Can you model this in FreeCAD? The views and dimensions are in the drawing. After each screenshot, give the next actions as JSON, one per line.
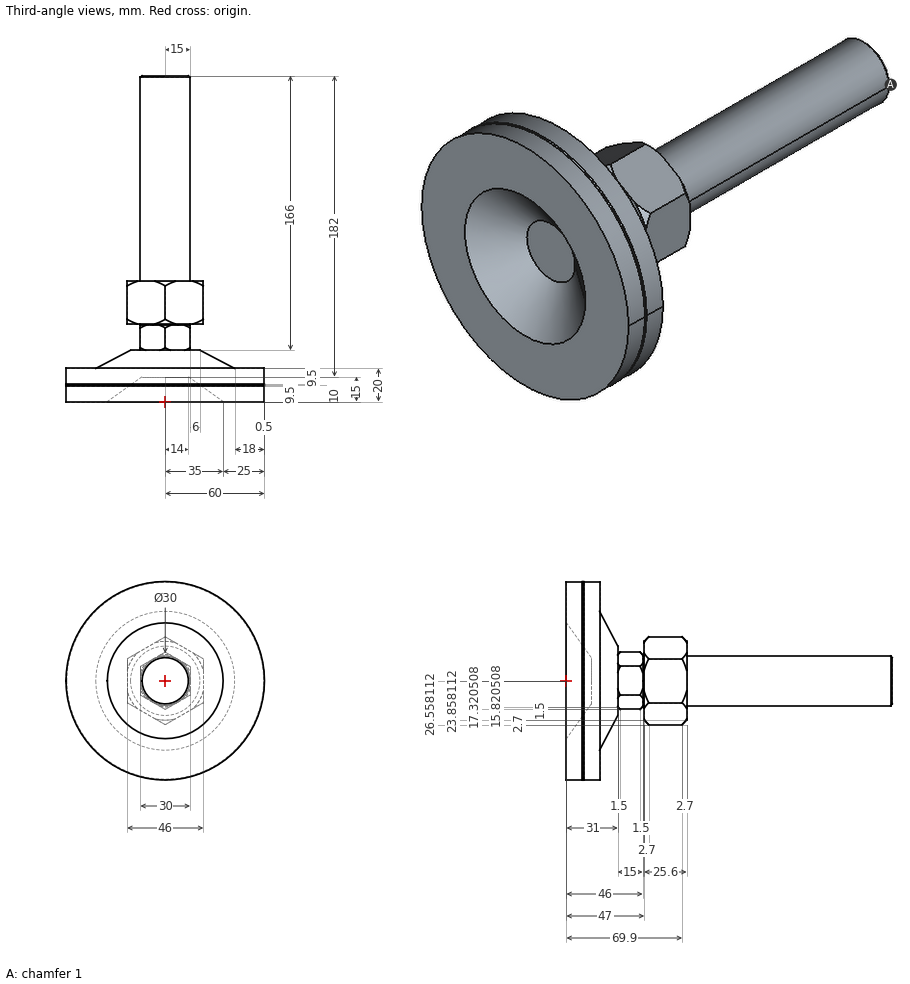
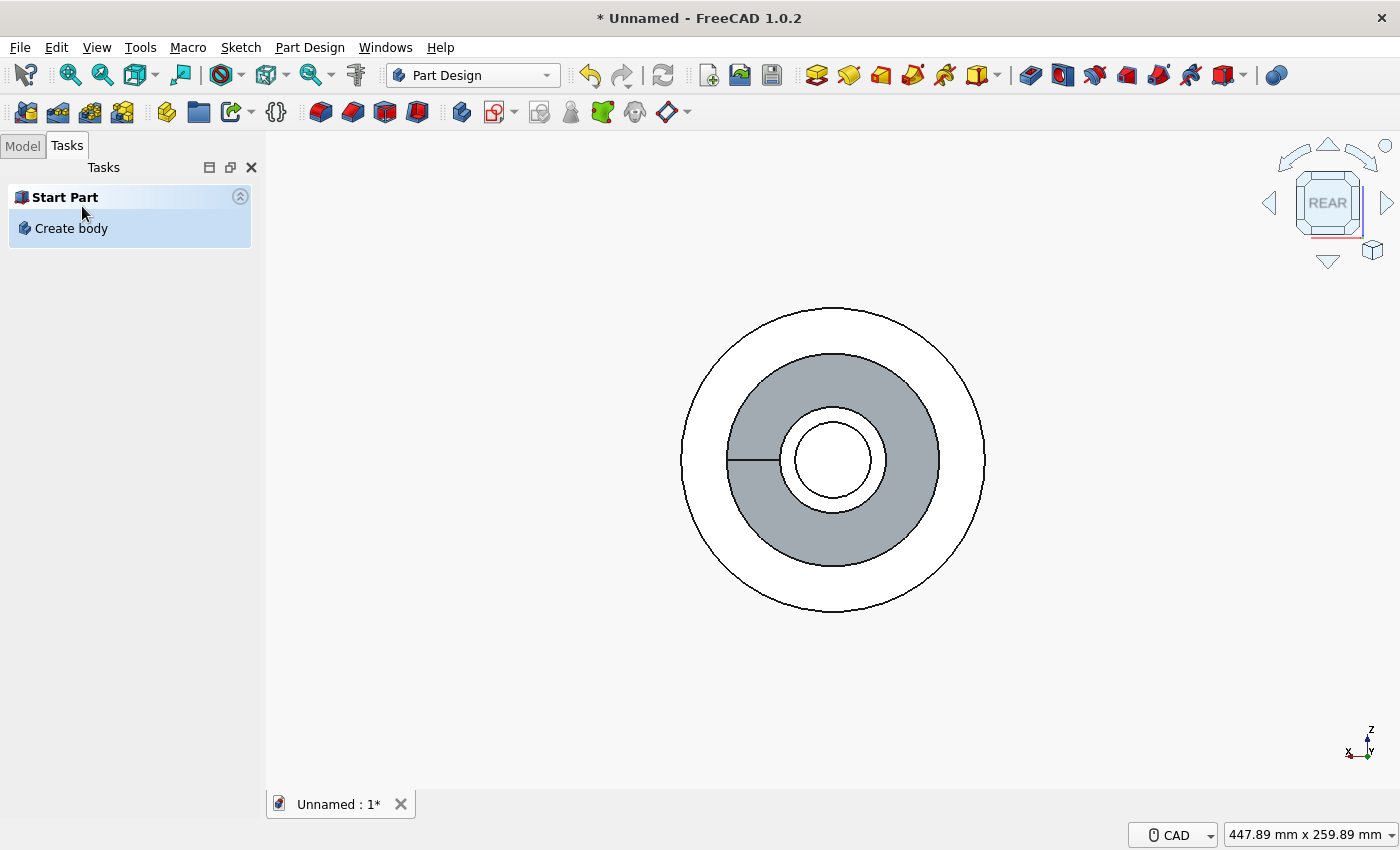
{"action": "key", "text": "2"}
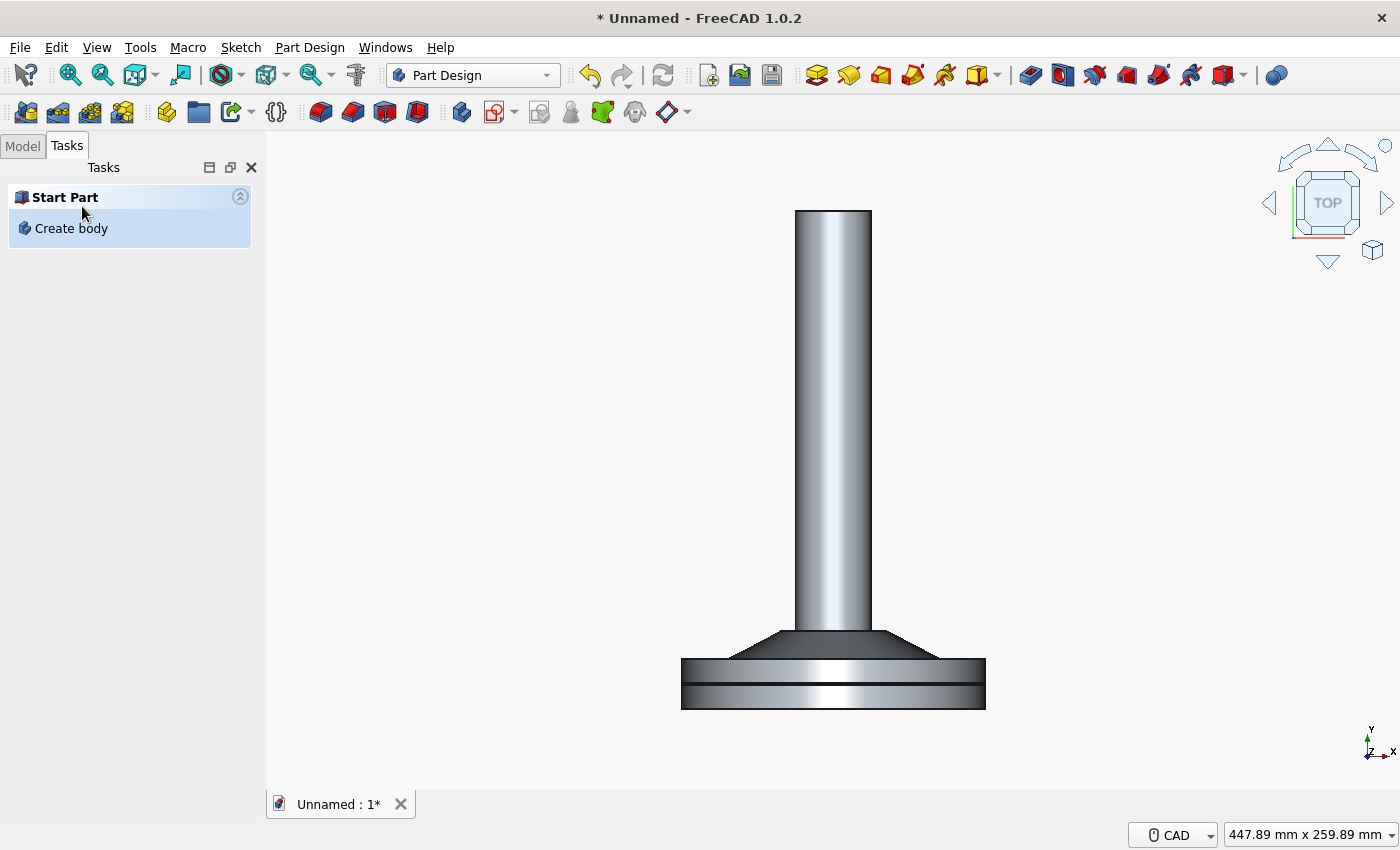
{"action": "key", "text": "3"}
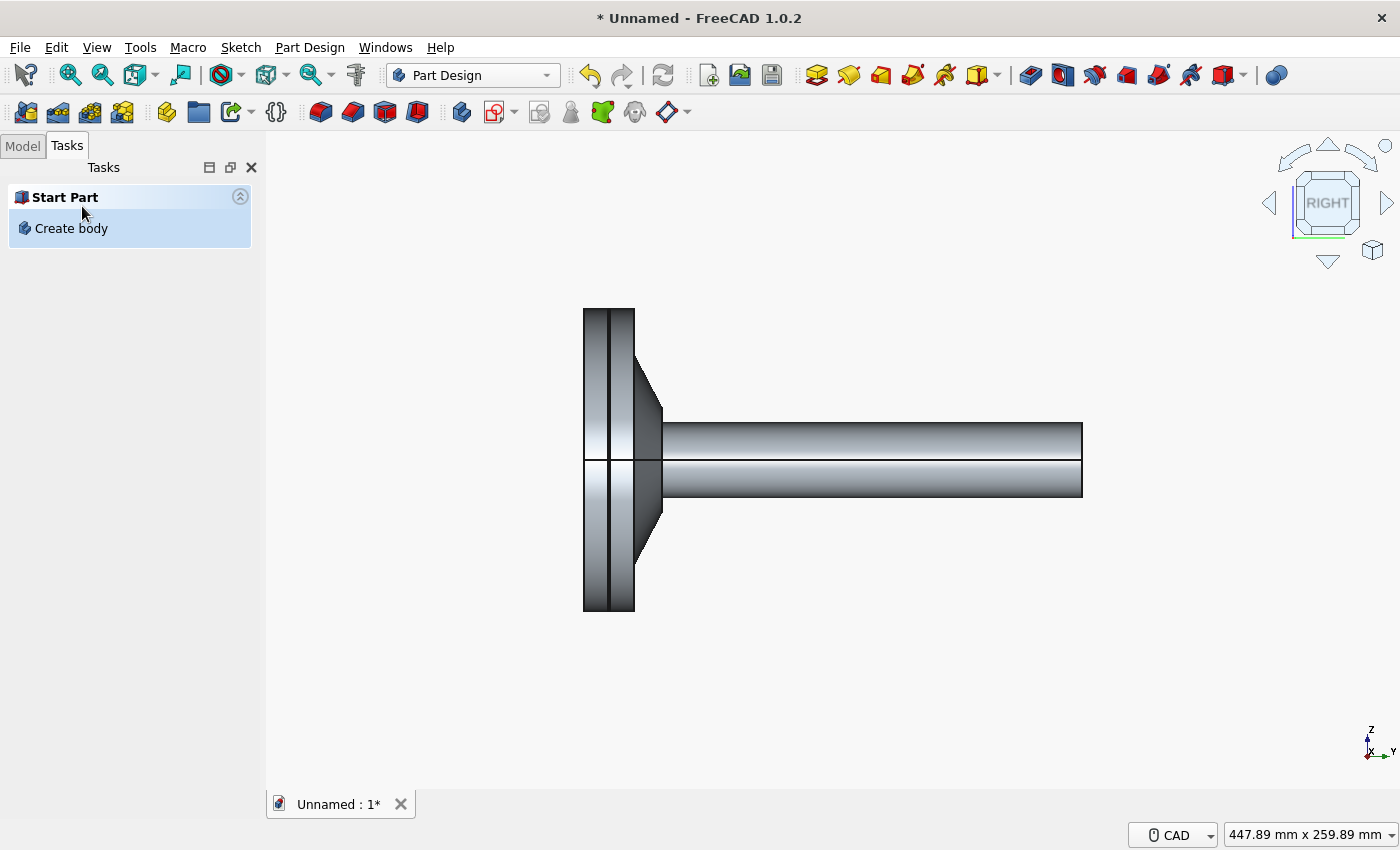
{"action": "left_click", "coordinate": [23, 145]}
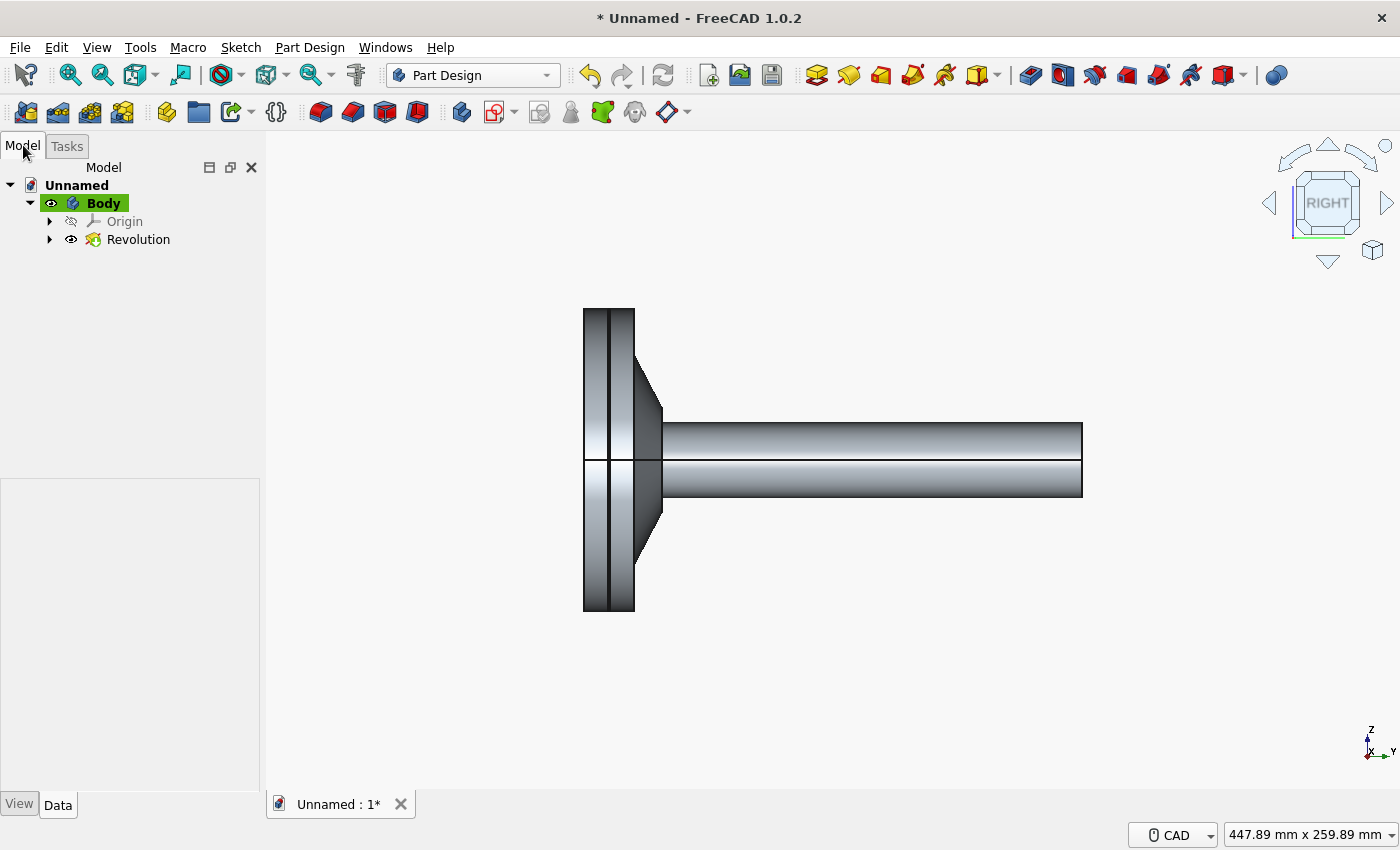
{"action": "left_click", "coordinate": [50, 221]}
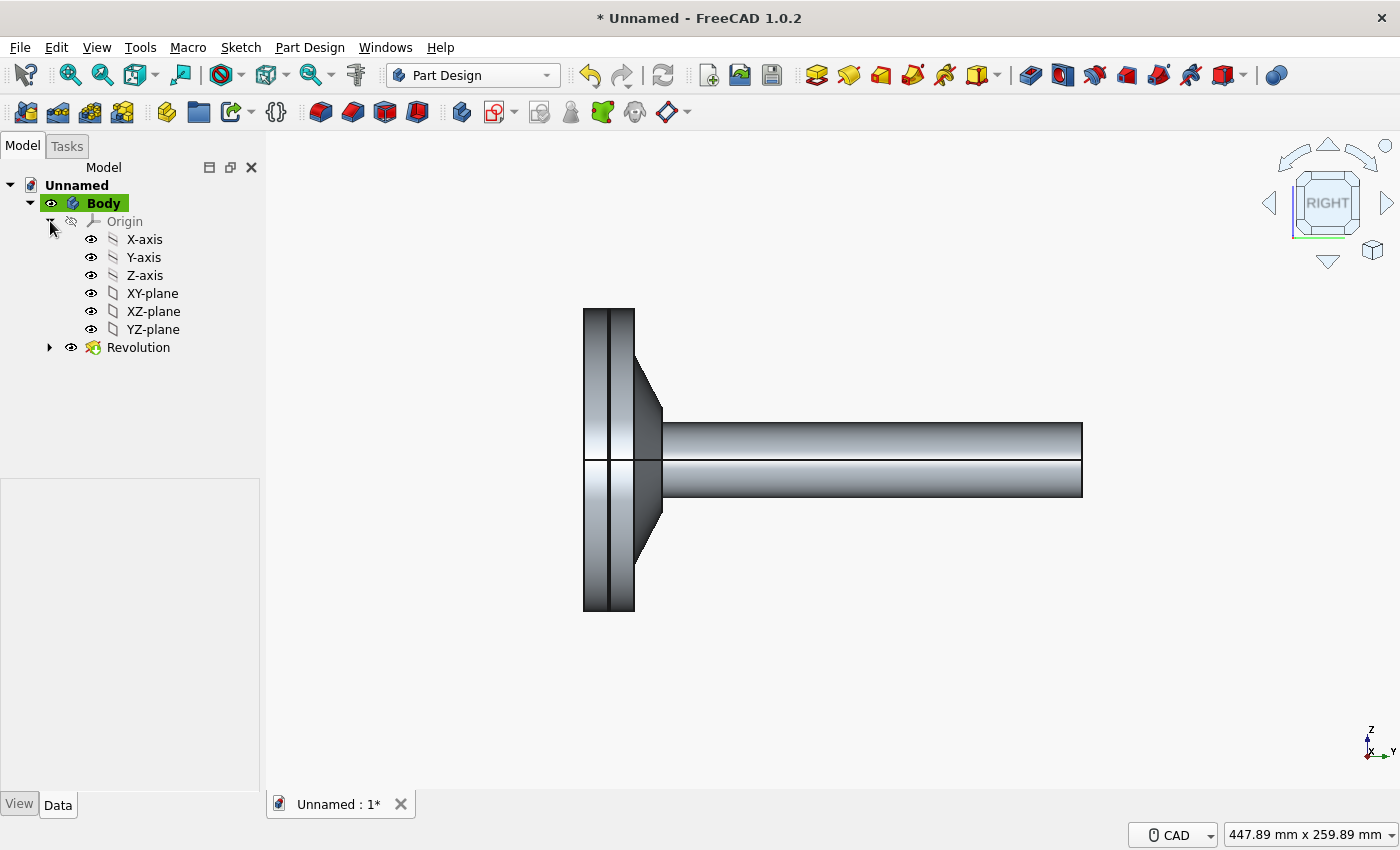
{"action": "left_click", "coordinate": [136, 311]}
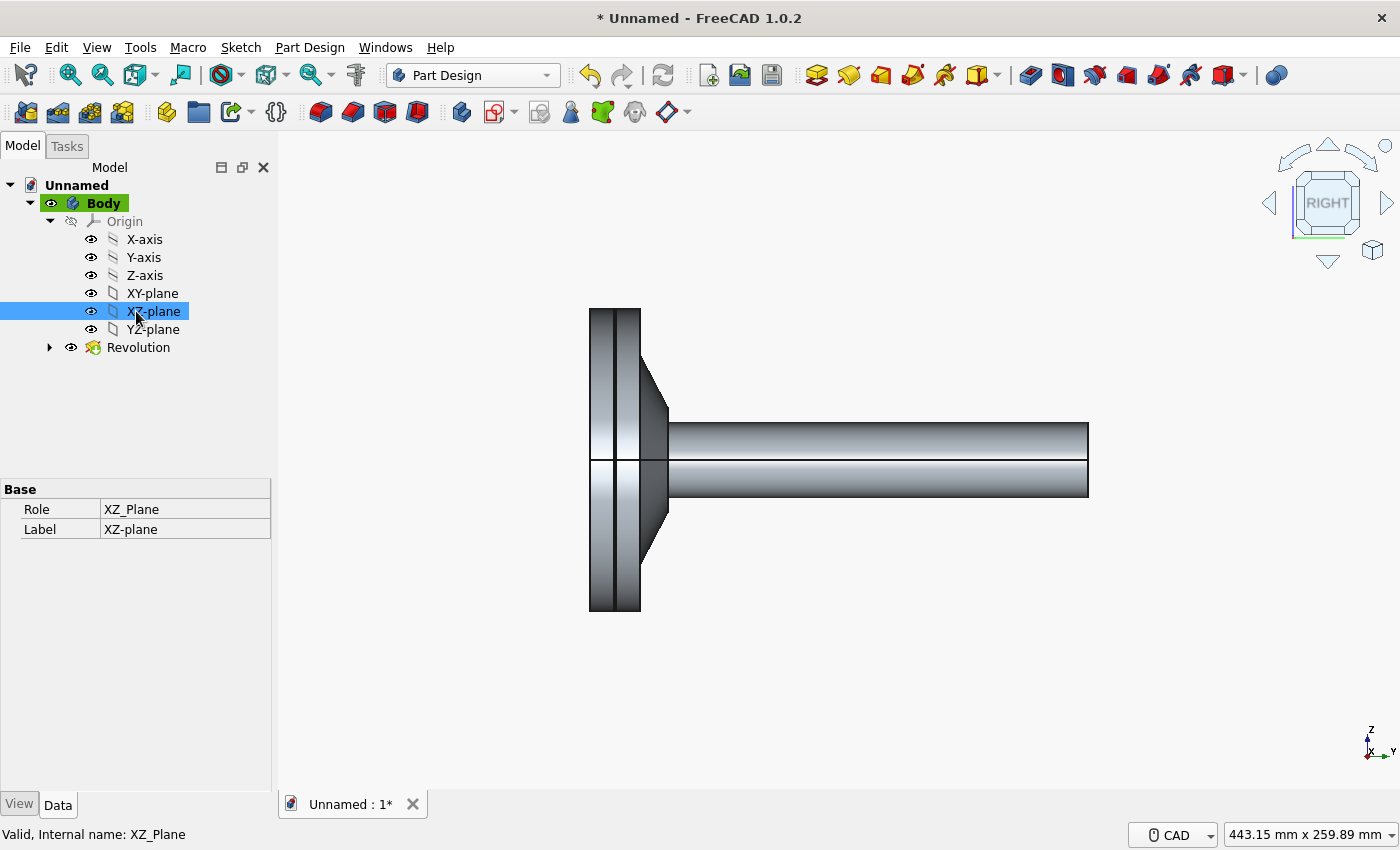
{"action": "left_click", "coordinate": [668, 112]}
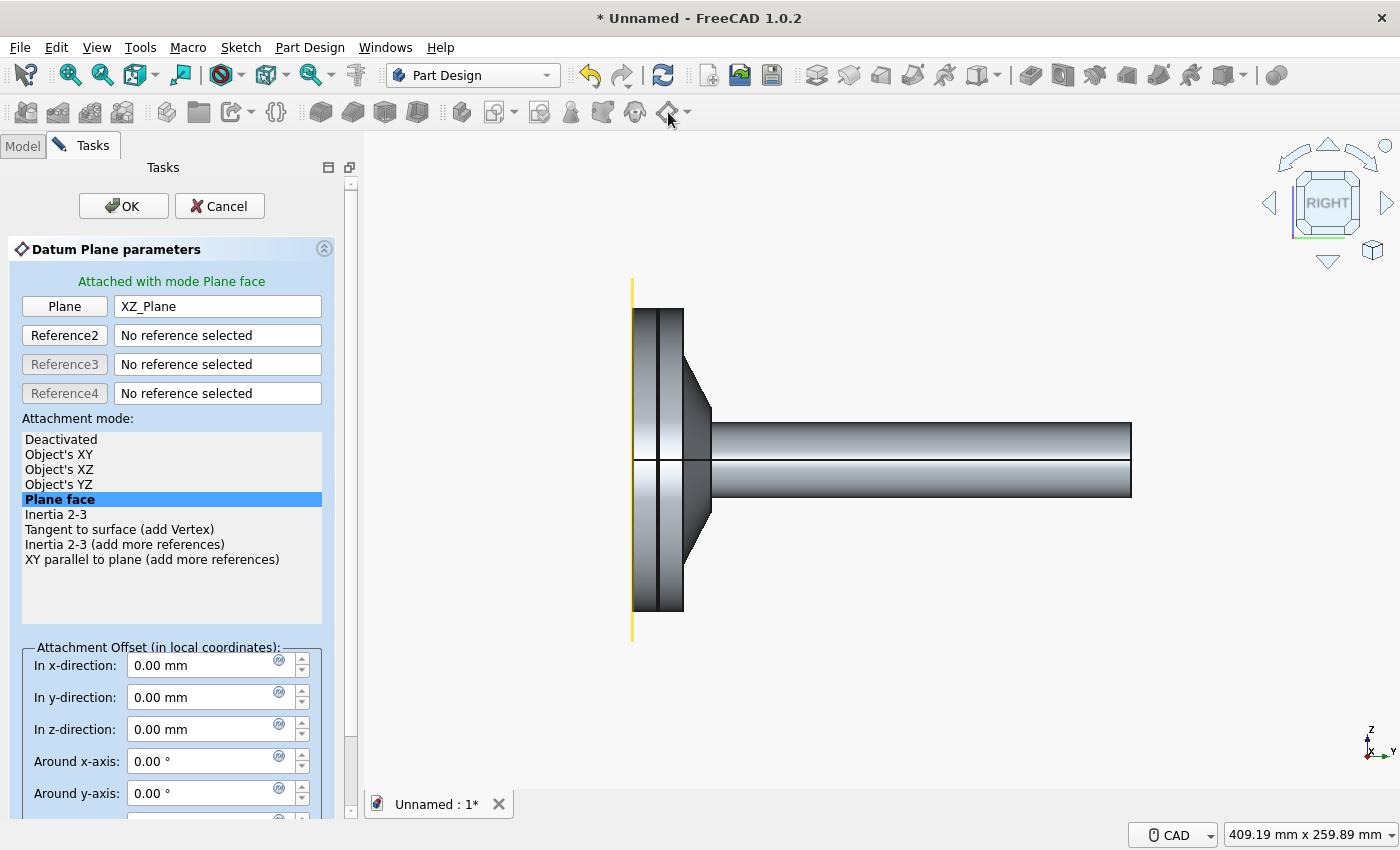
{"action": "triple_click", "coordinate": [210, 729]}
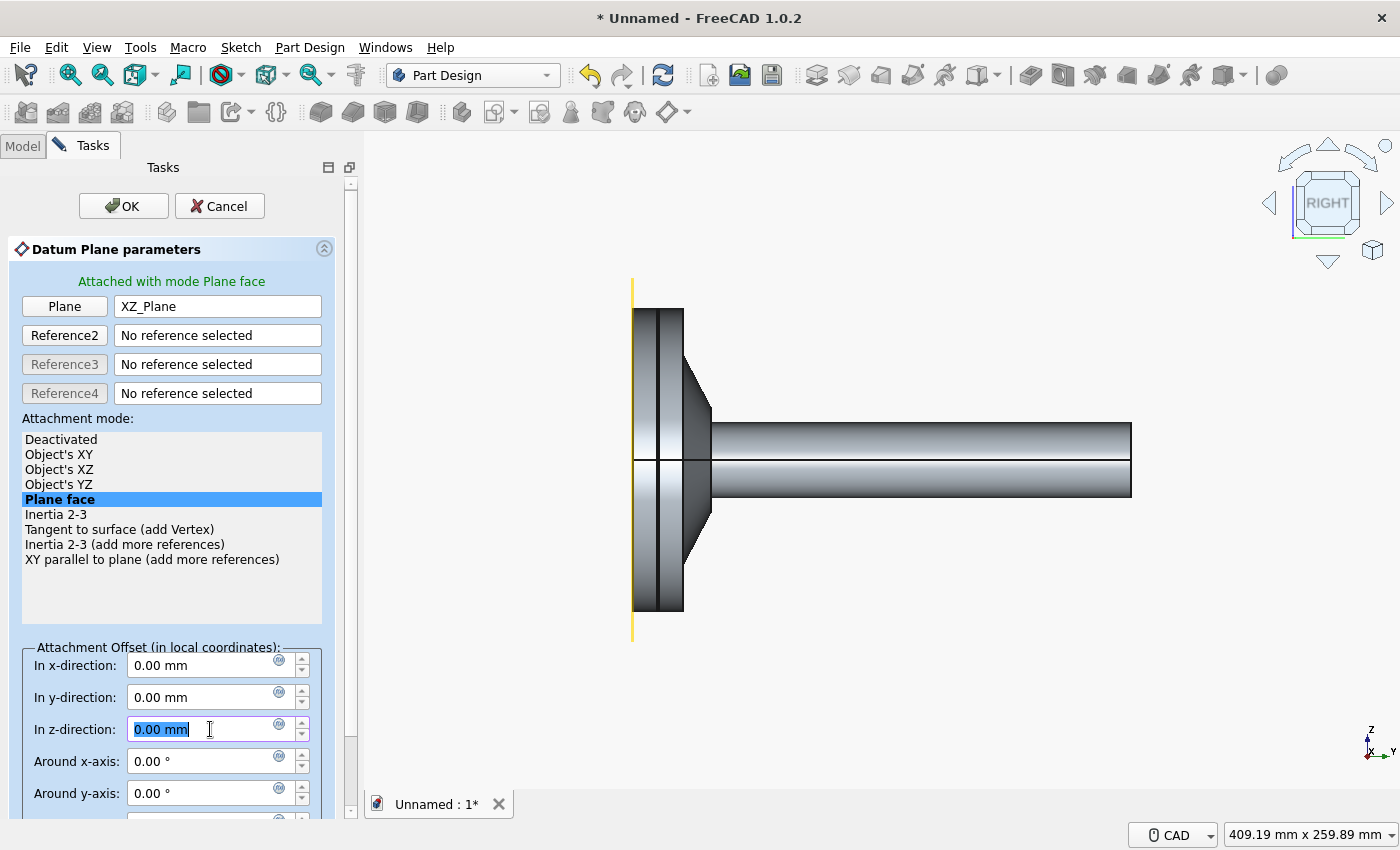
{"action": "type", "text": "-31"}
{"action": "key", "text": "Tab"}